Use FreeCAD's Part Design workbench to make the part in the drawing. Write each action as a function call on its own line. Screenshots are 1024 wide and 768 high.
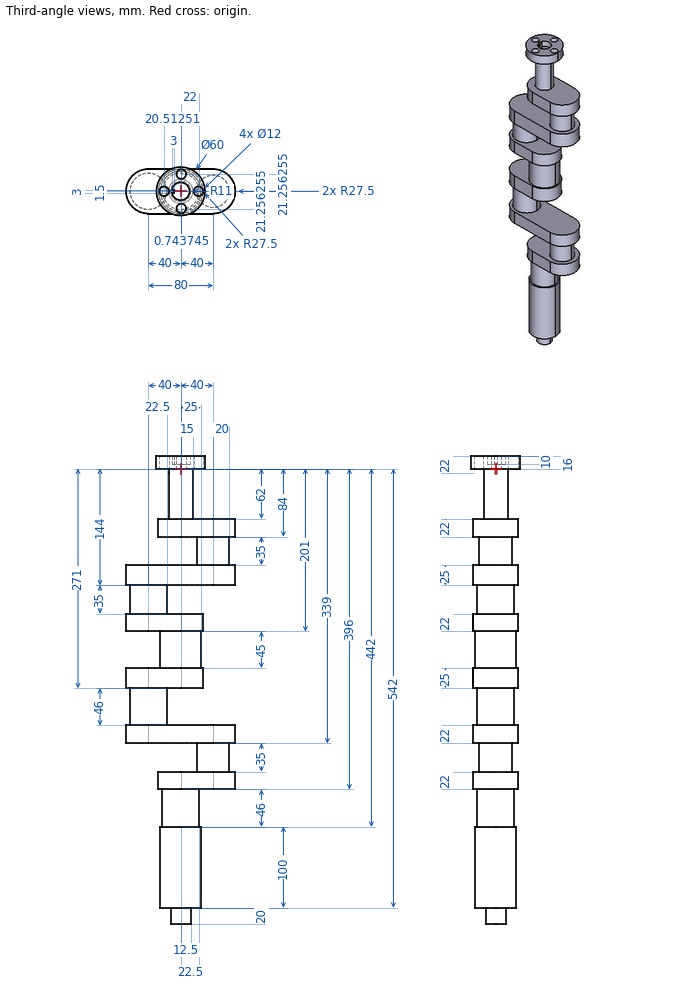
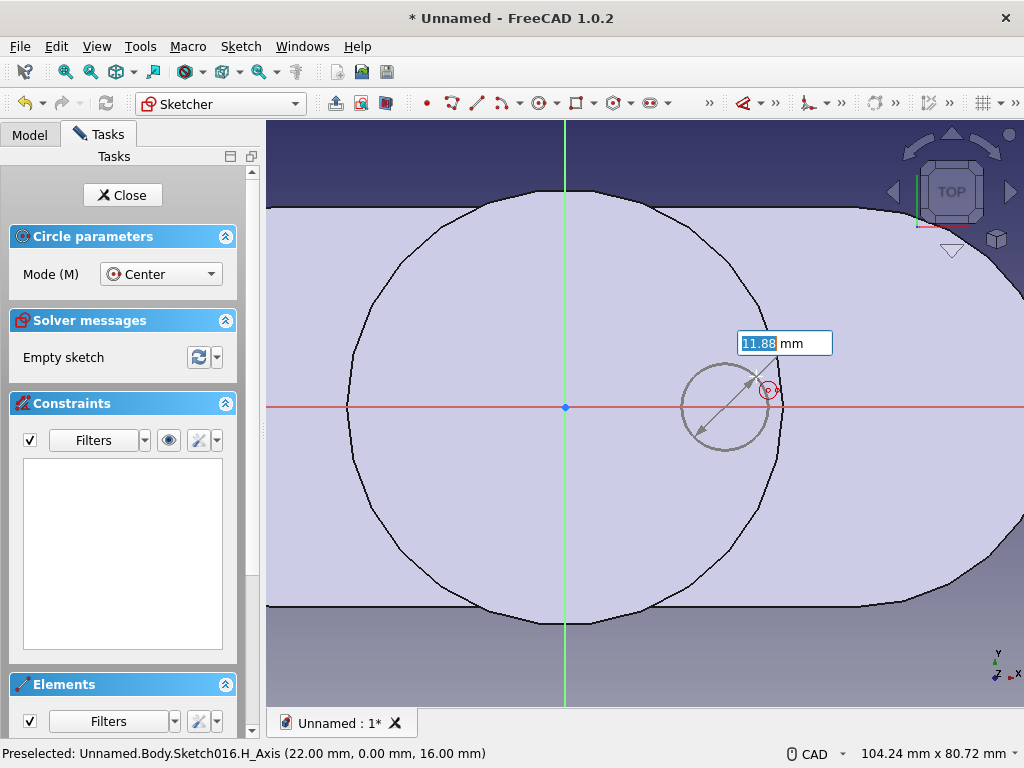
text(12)
key(Return)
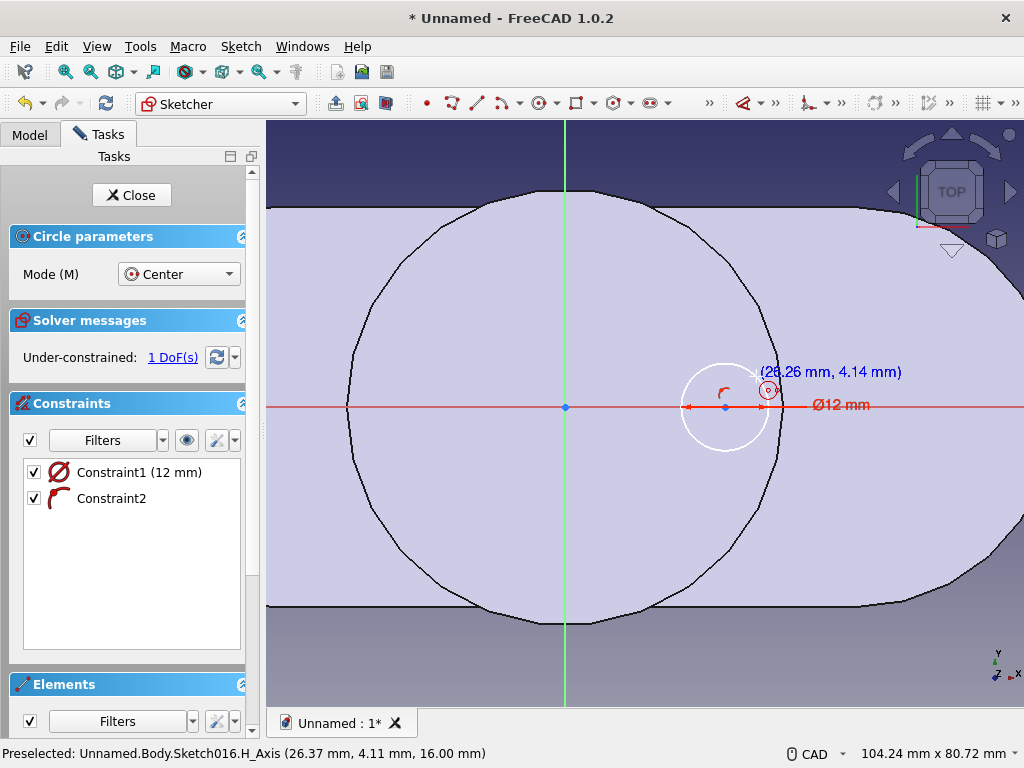
scroll(570, 562, up, 6)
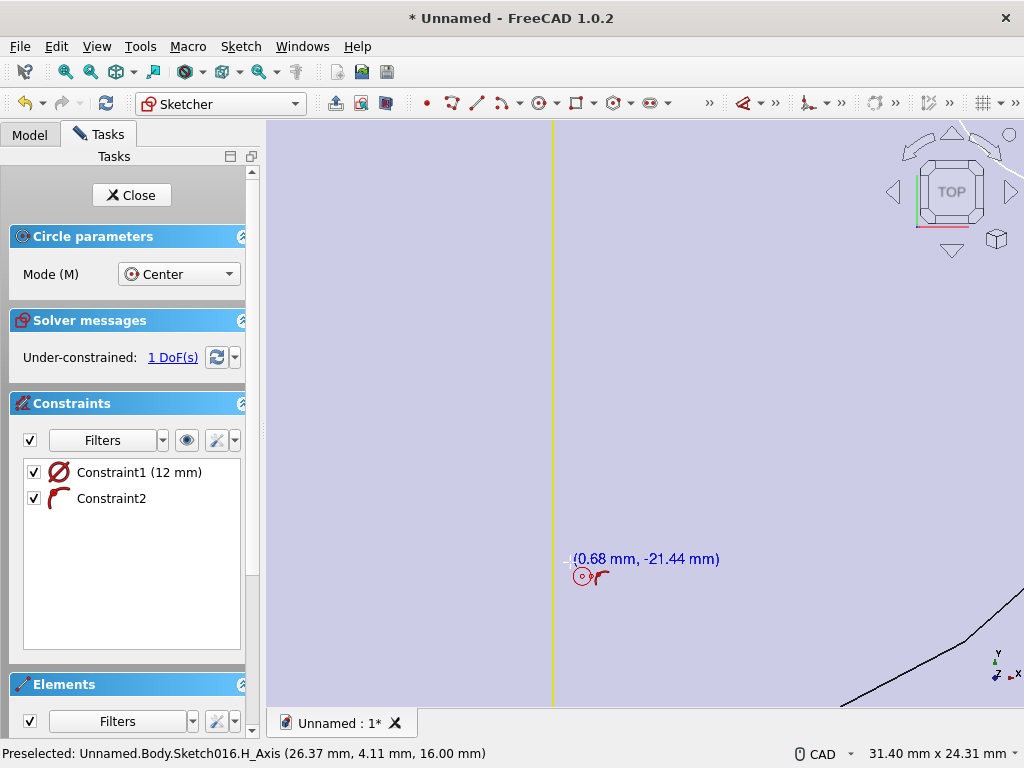
click(571, 559)
move(673, 457)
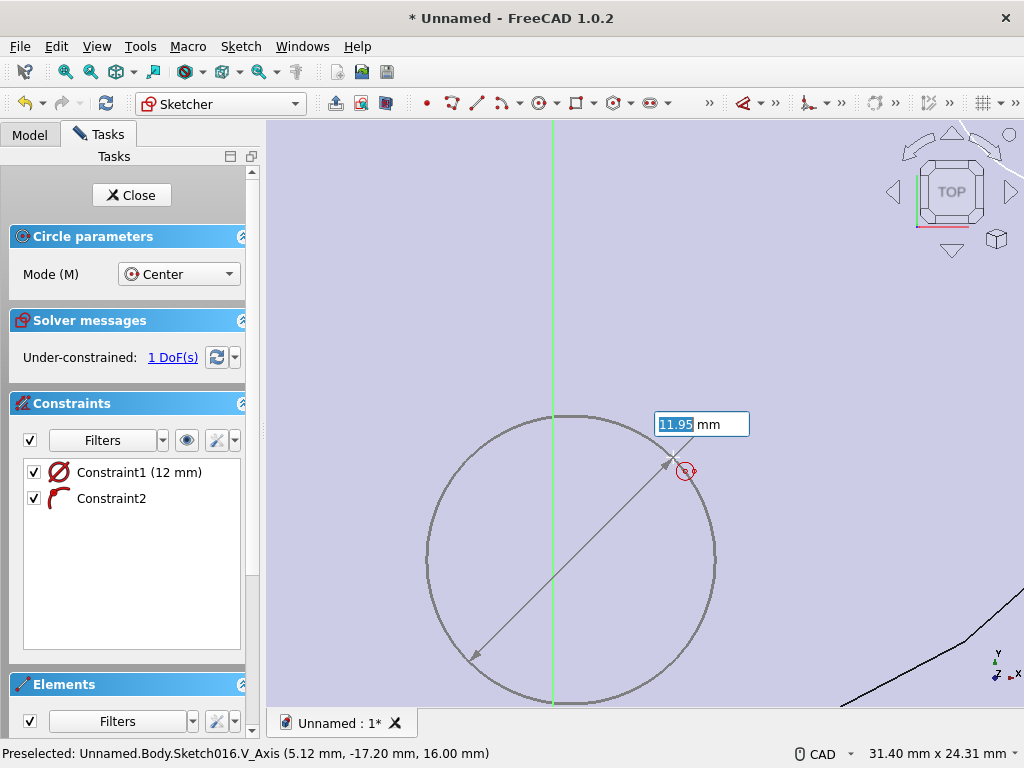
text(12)
key(Return)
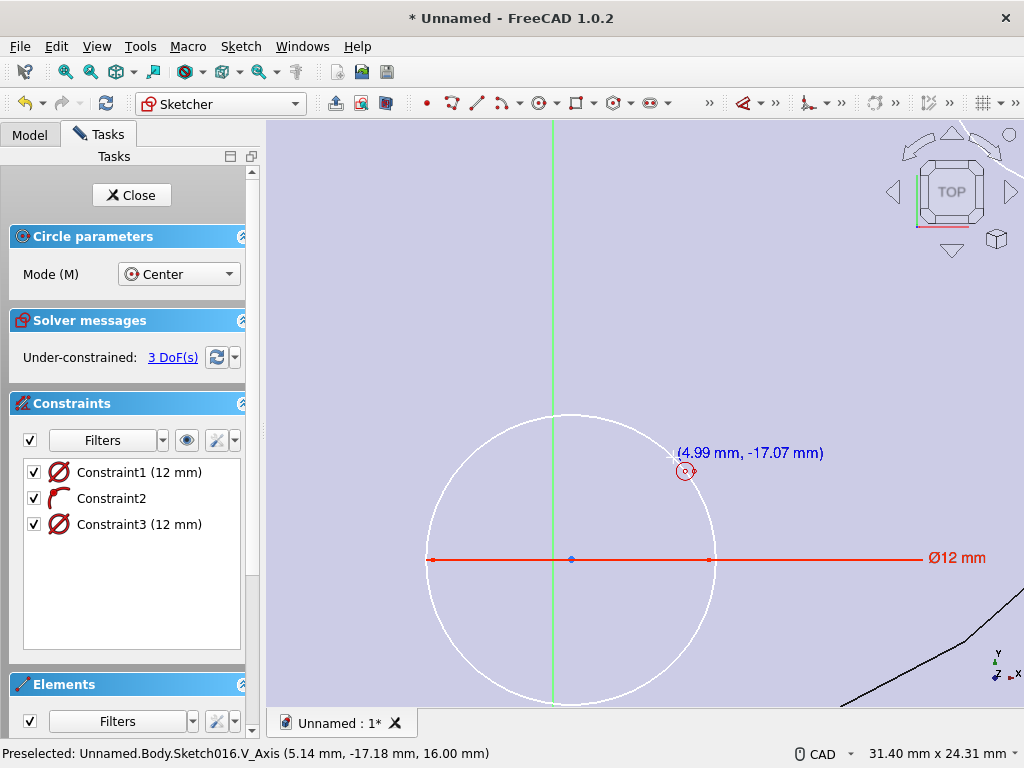
scroll(579, 572, down, 6)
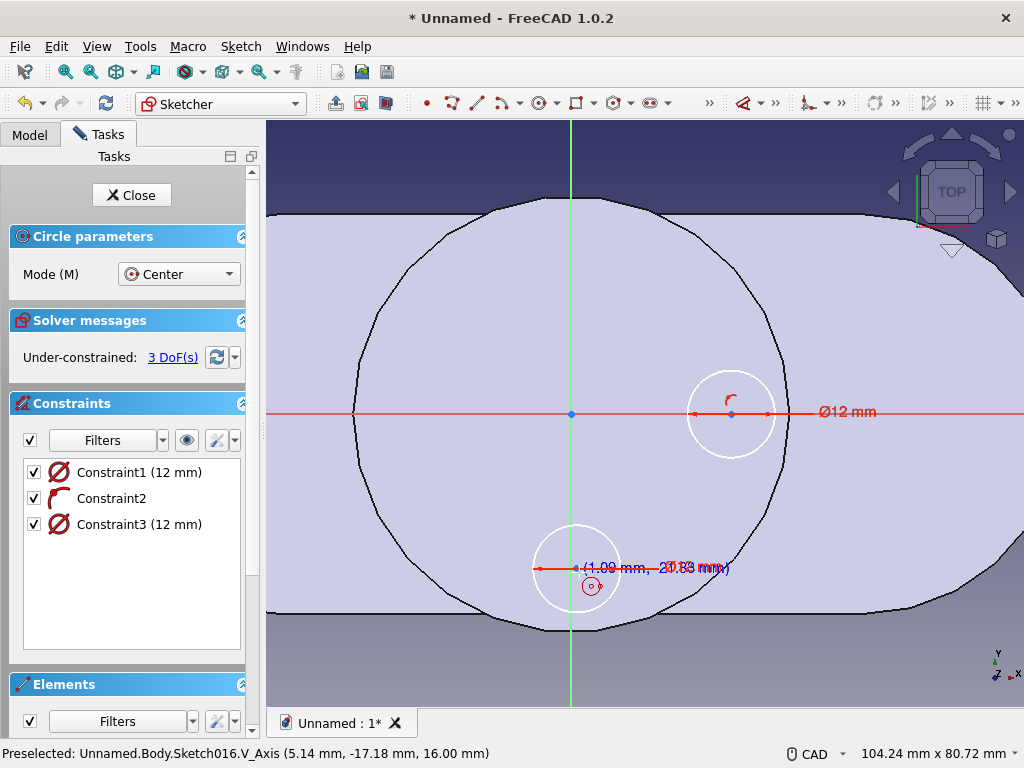
click(422, 414)
move(453, 383)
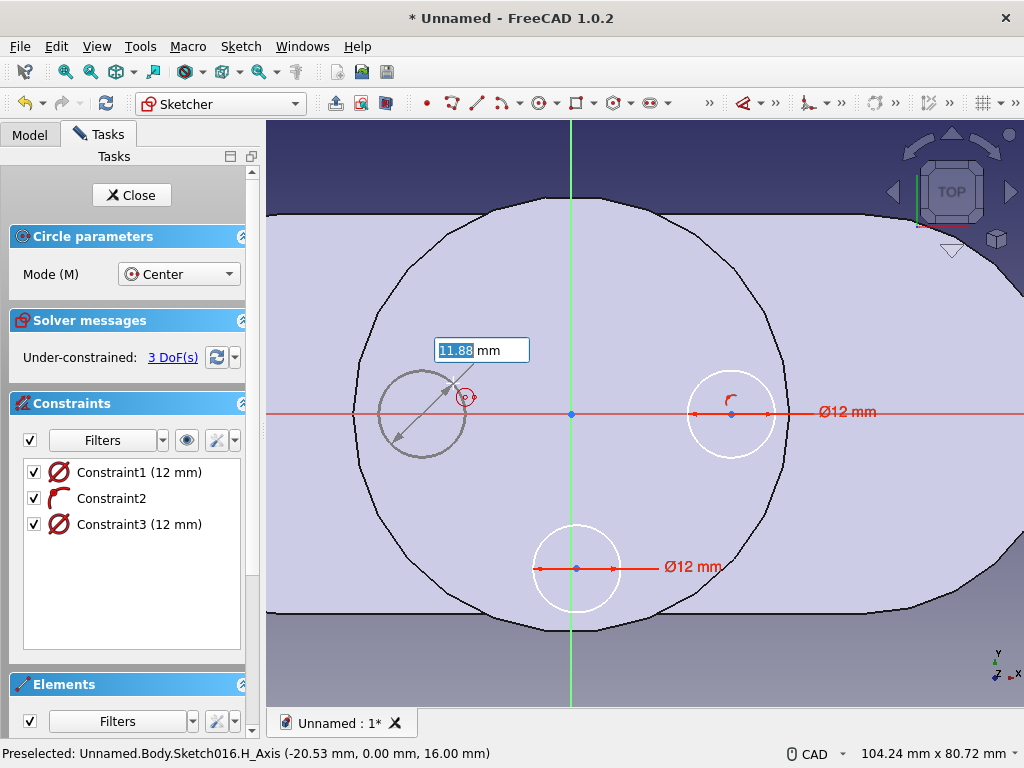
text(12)
key(Return)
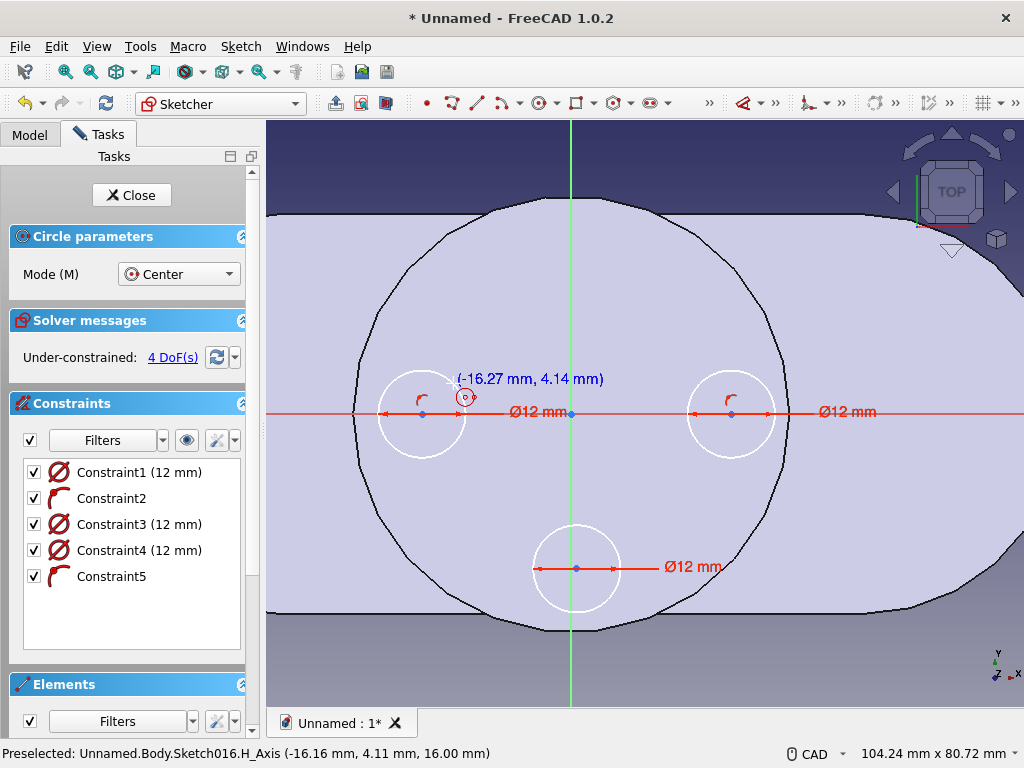
scroll(577, 260, up, 6)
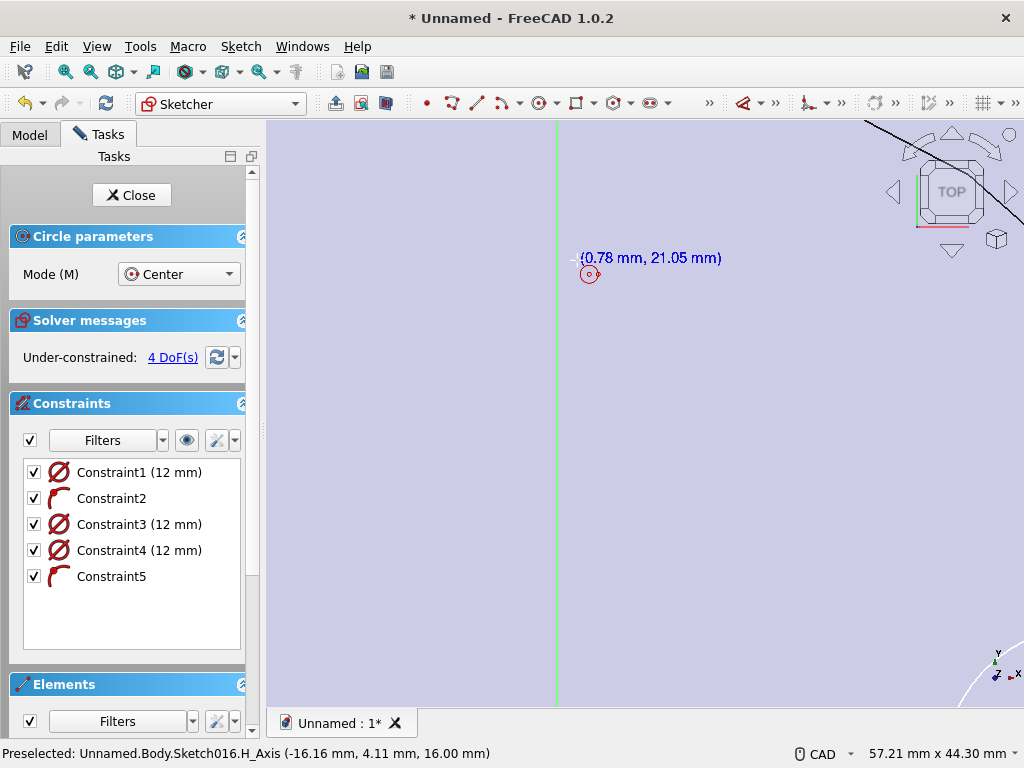
click(575, 258)
move(678, 155)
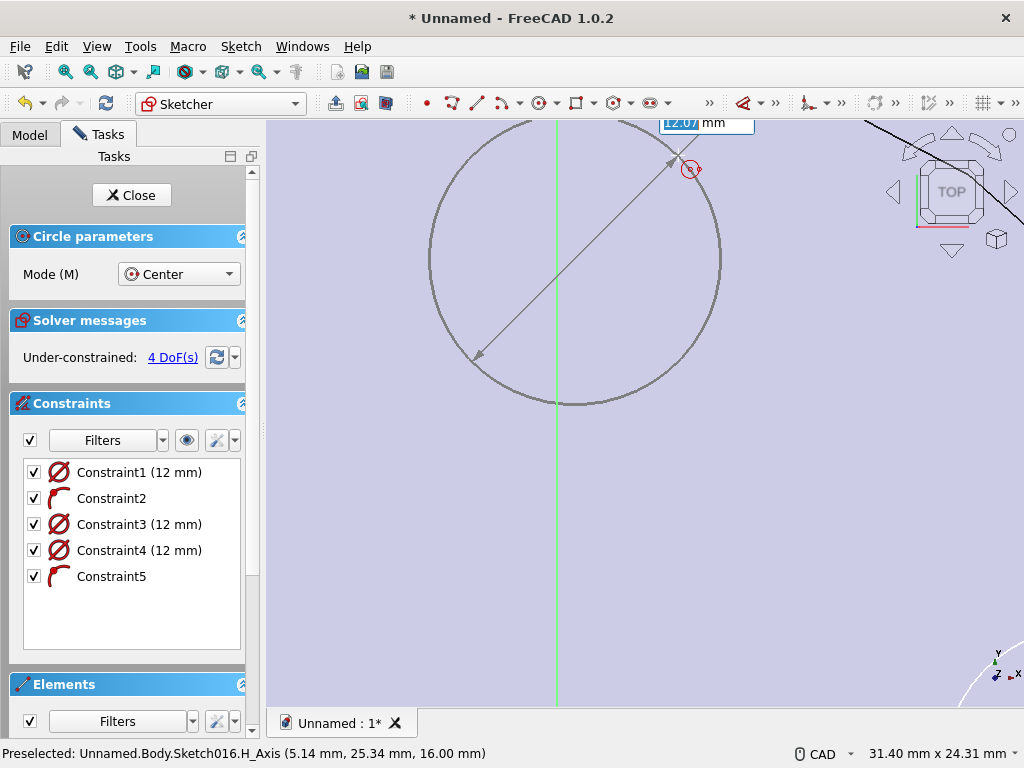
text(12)
key(Return)
key(Escape)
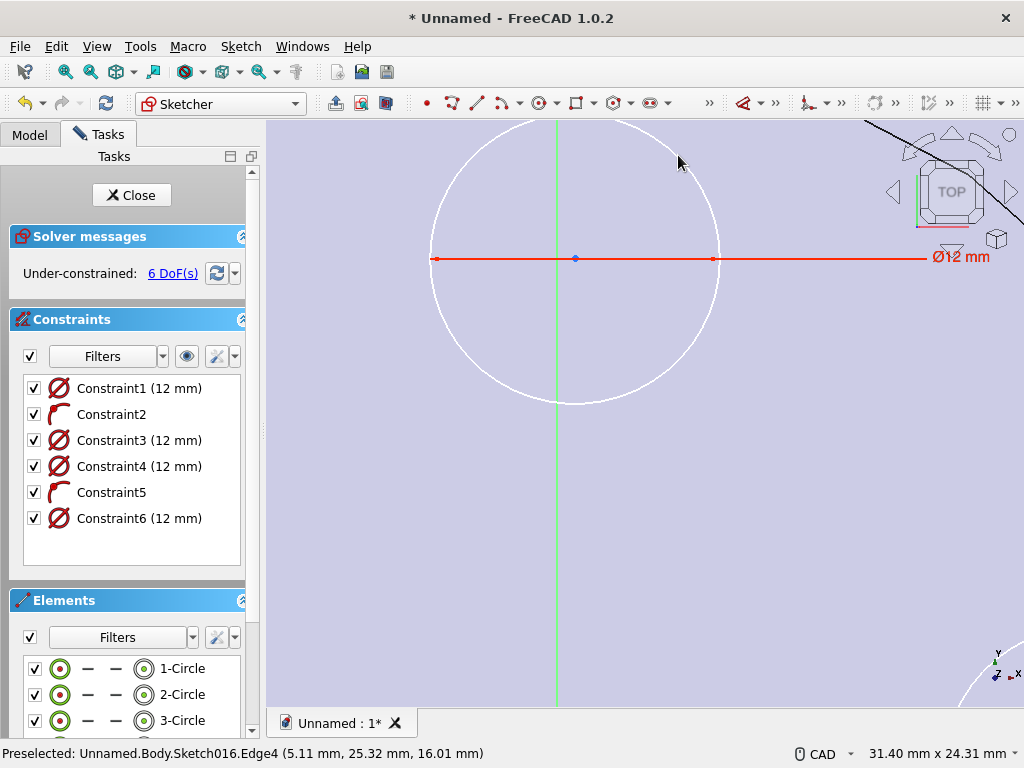
scroll(577, 259, down, 6)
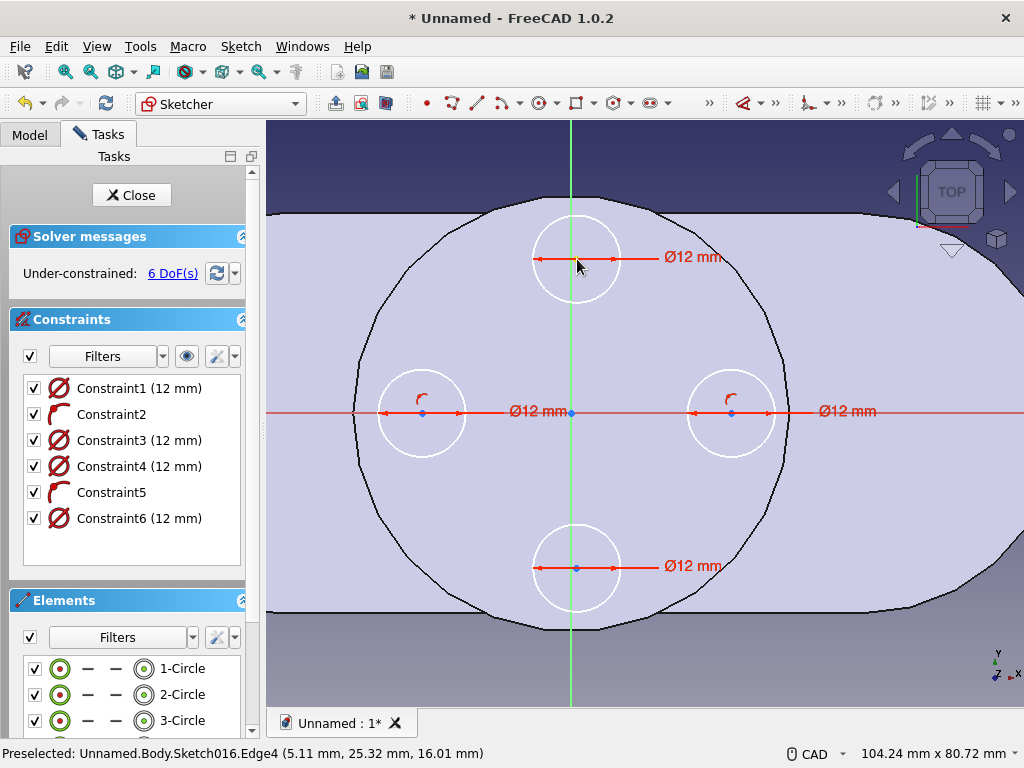
click(577, 568)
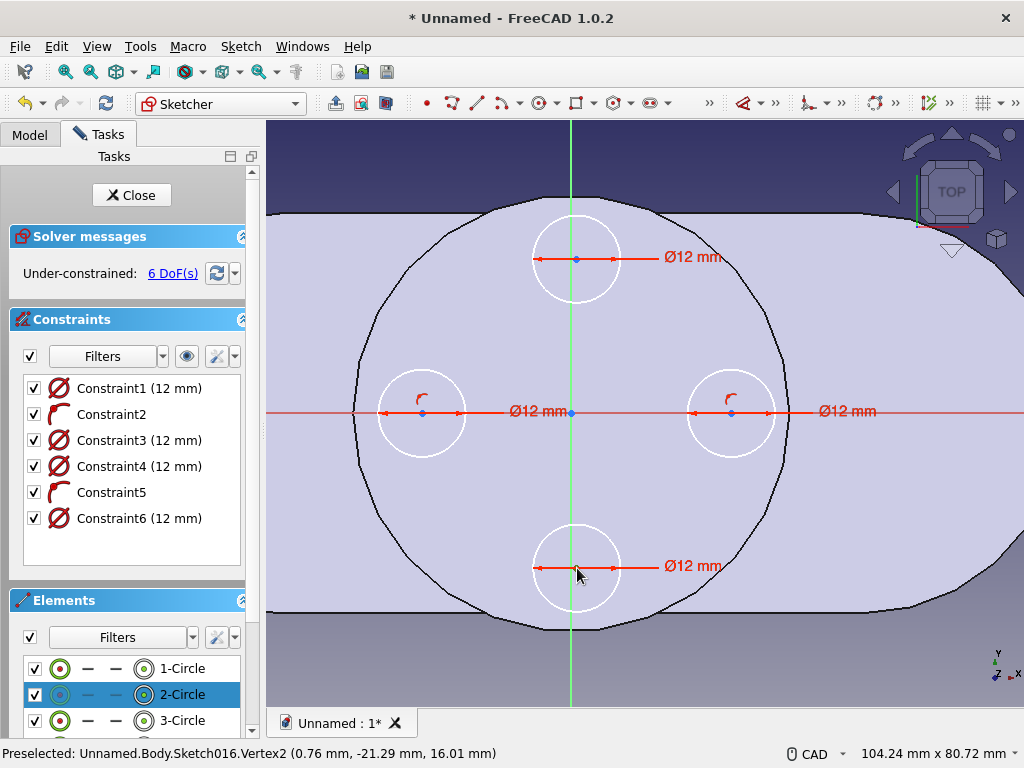
click(577, 259)